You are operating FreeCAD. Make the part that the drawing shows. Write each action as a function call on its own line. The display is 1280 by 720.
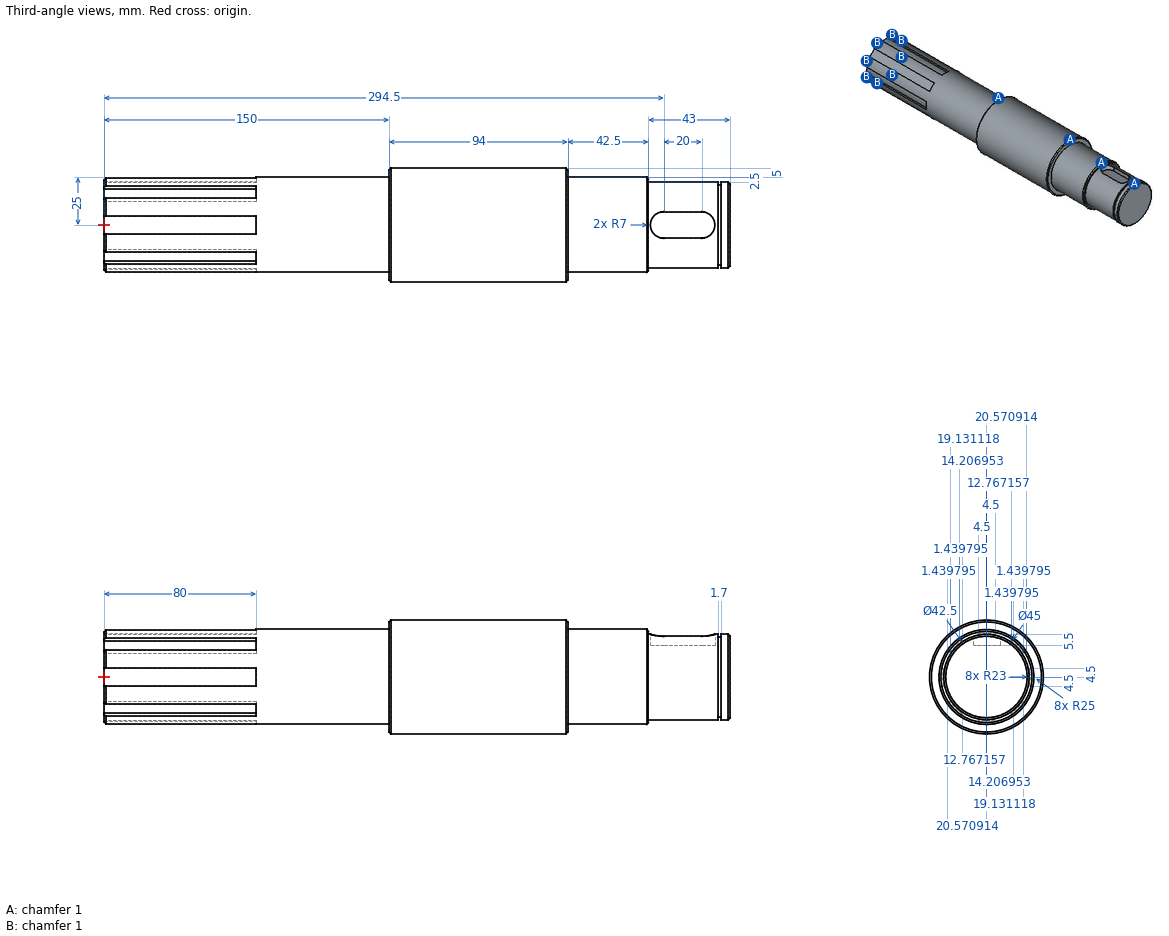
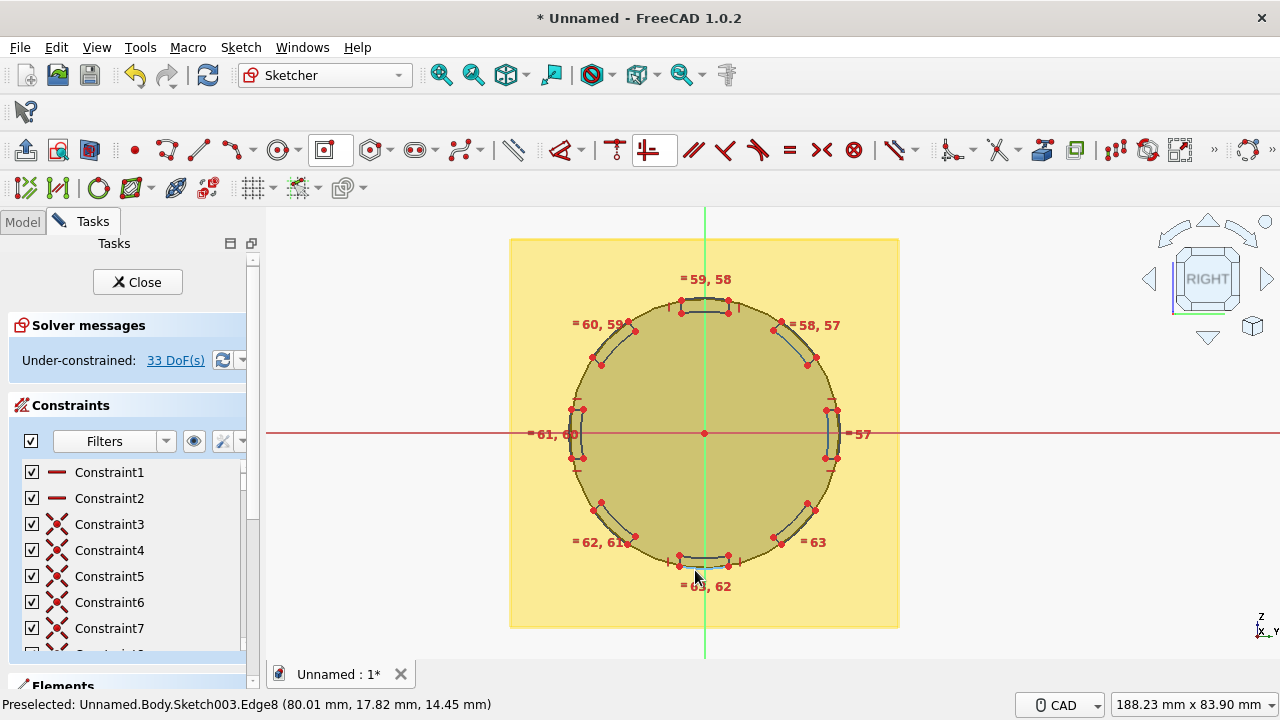
scroll(714, 312, up, 2)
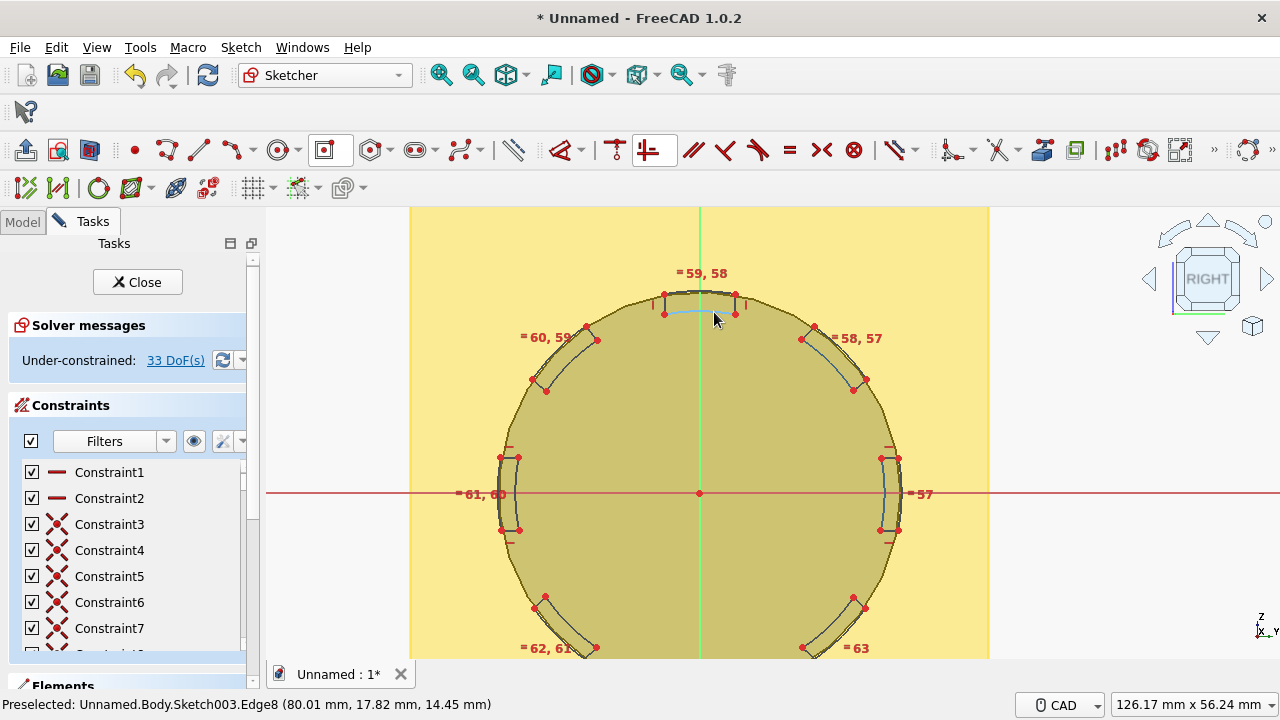
click(714, 312)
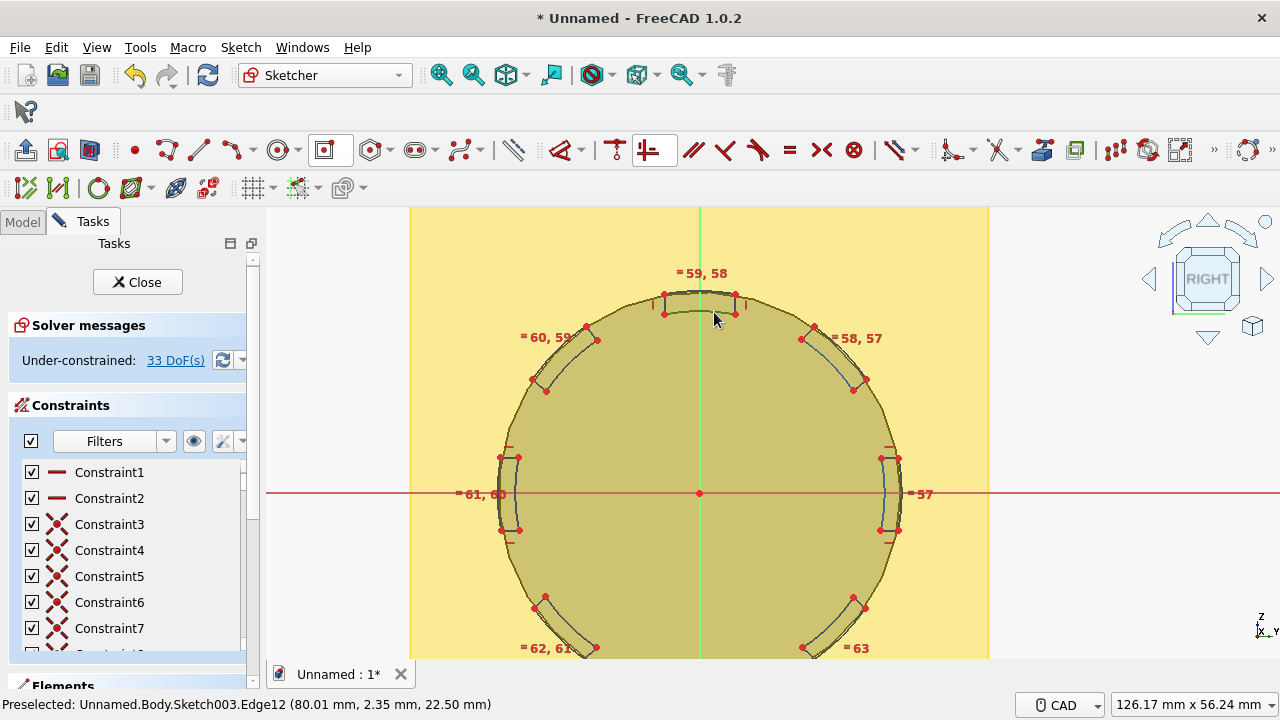
click(580, 354)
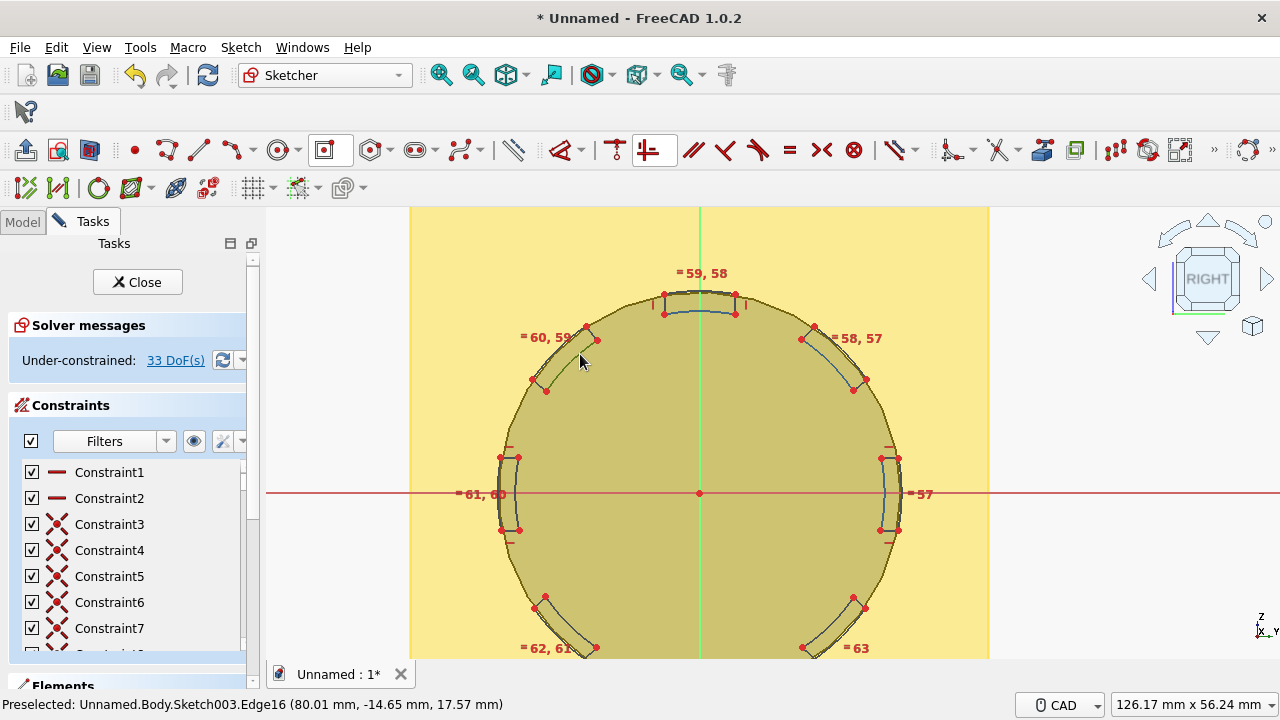
click(516, 480)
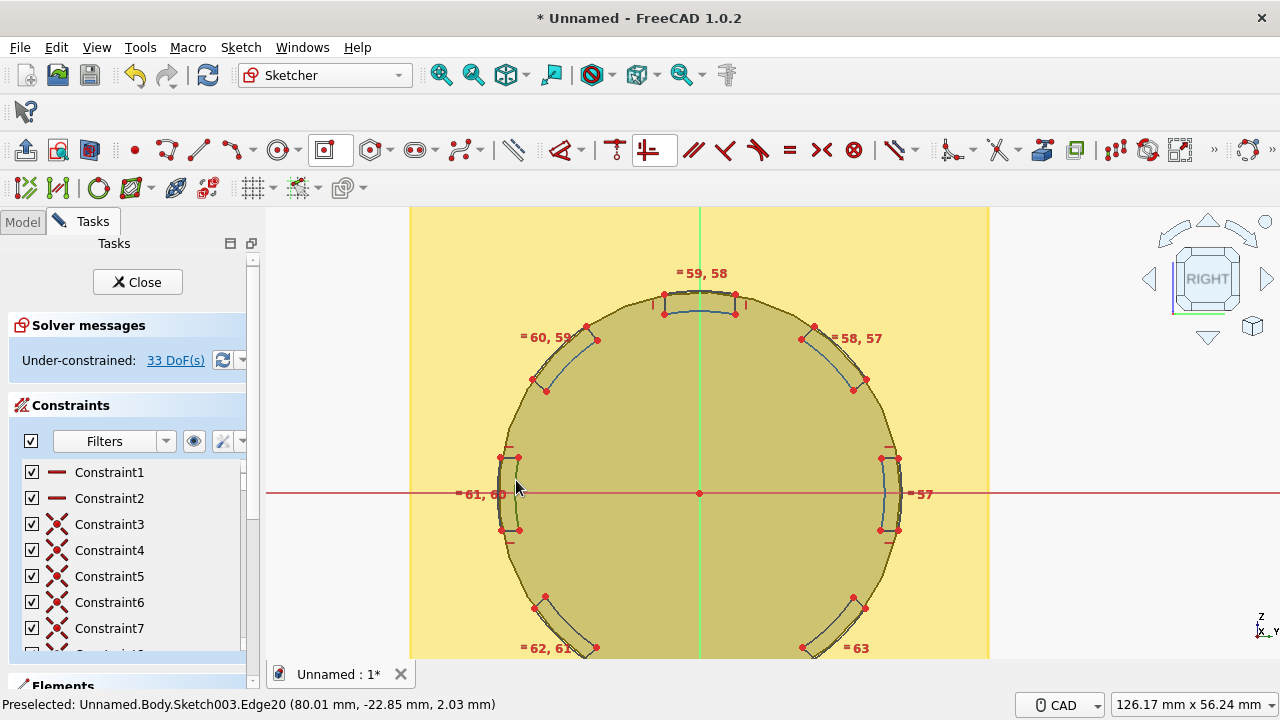
click(559, 614)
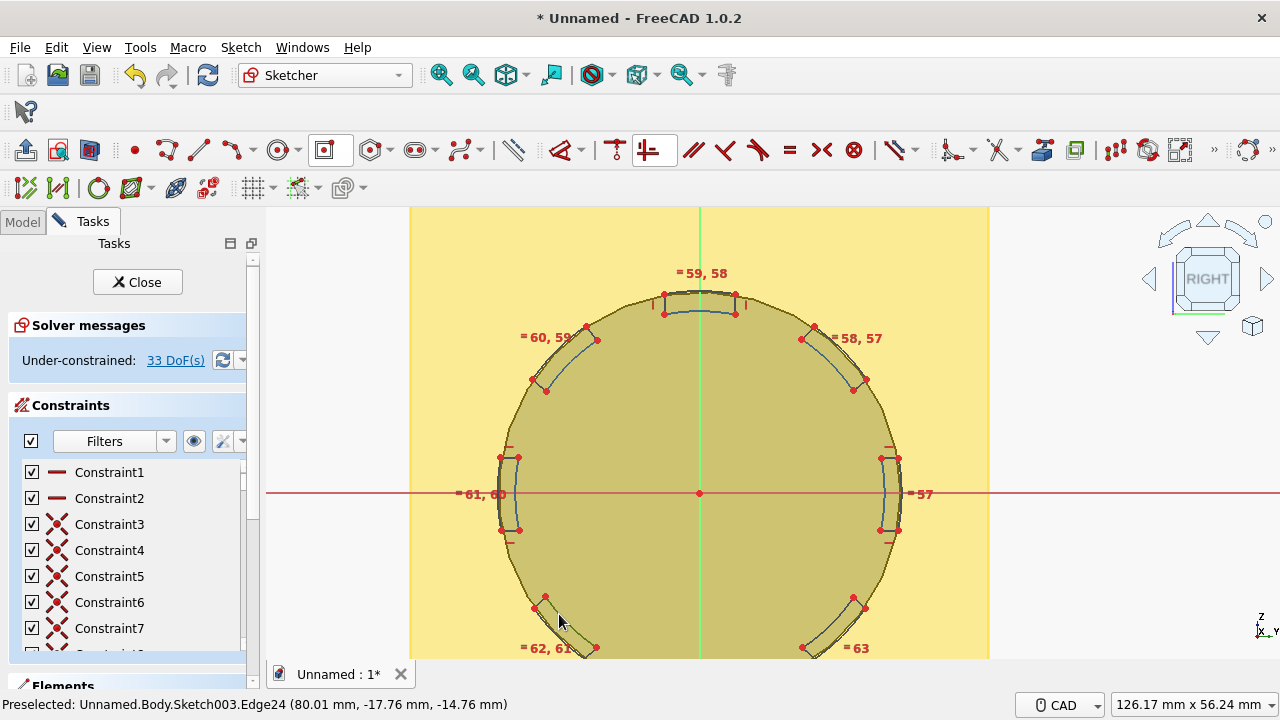
scroll(714, 311, down, 2)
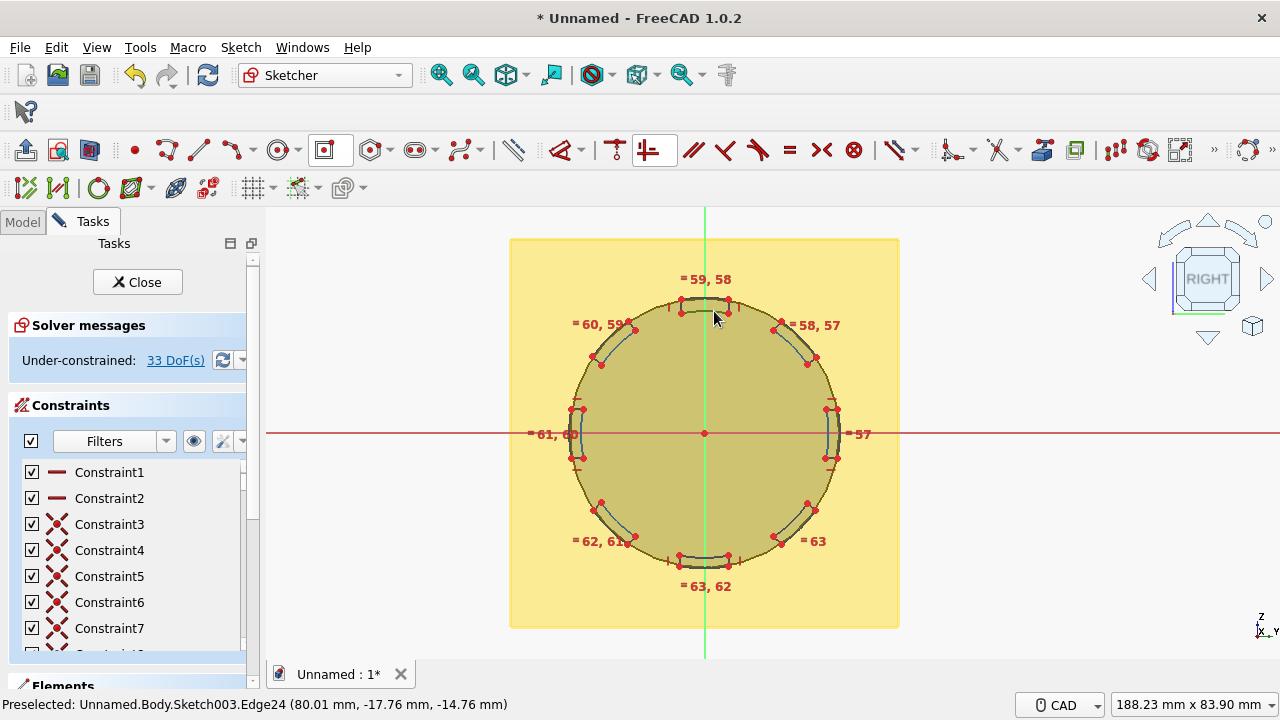
scroll(695, 557, up, 2)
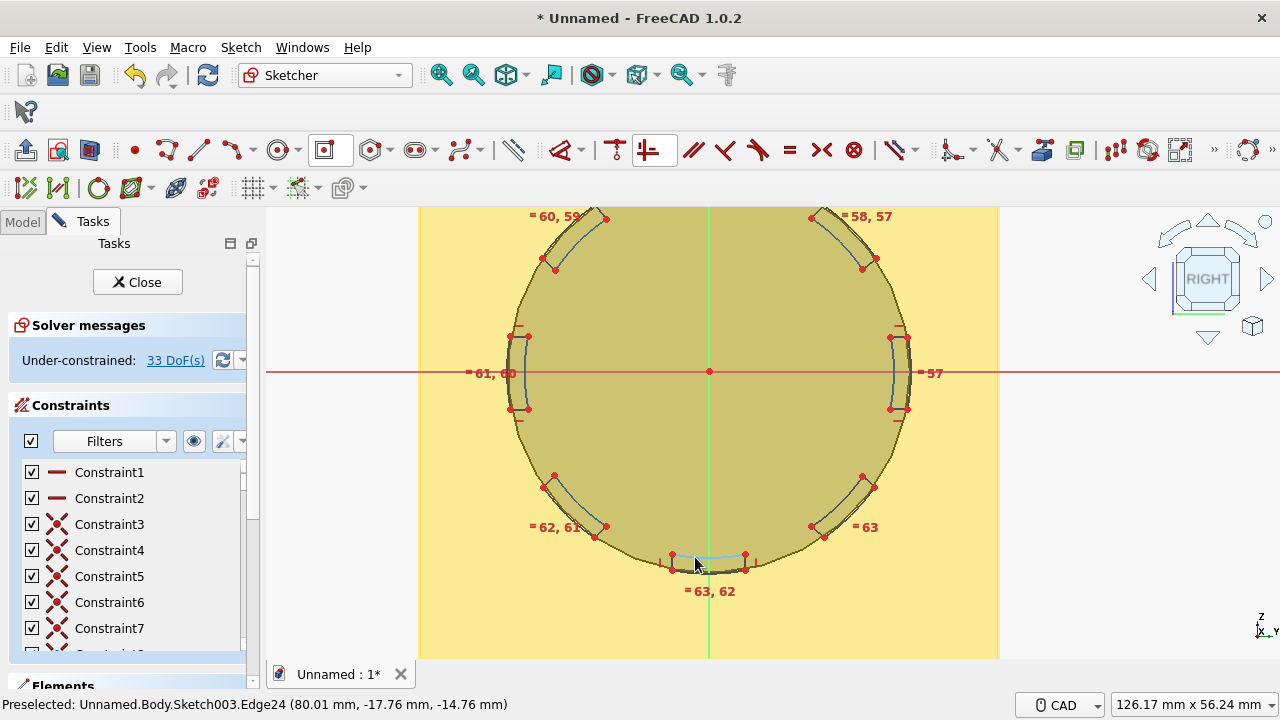
click(694, 557)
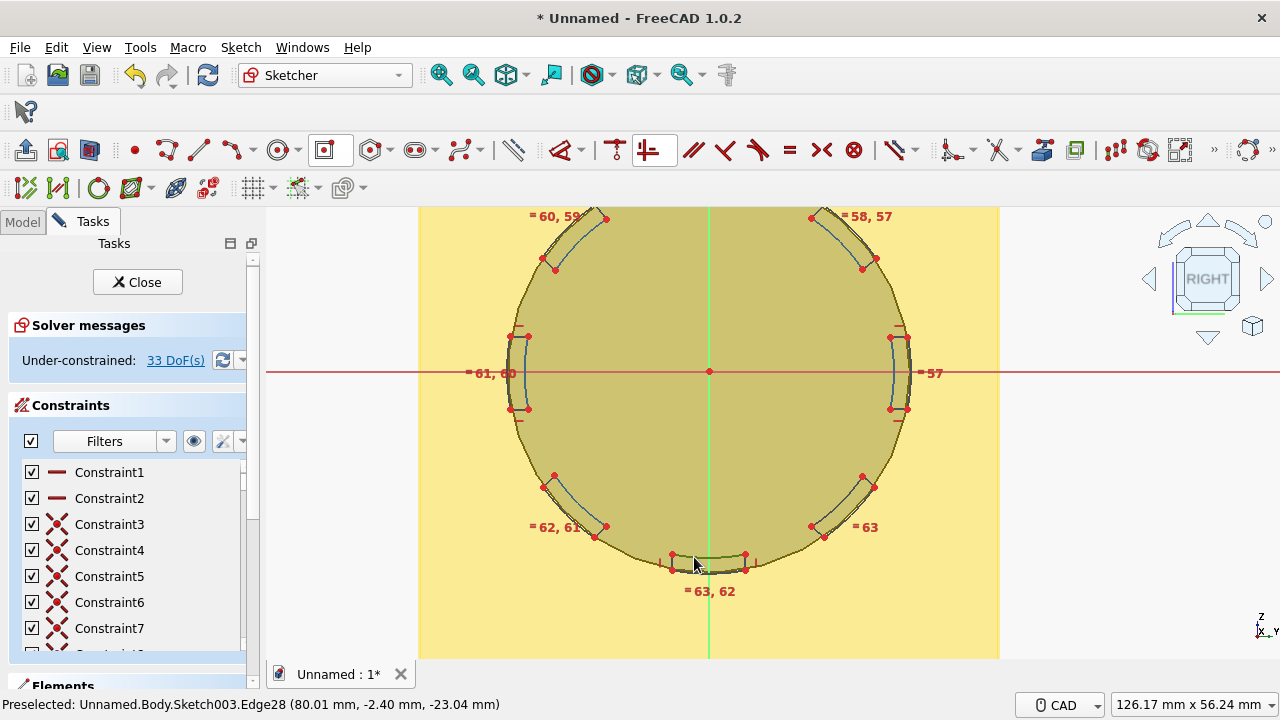
click(829, 514)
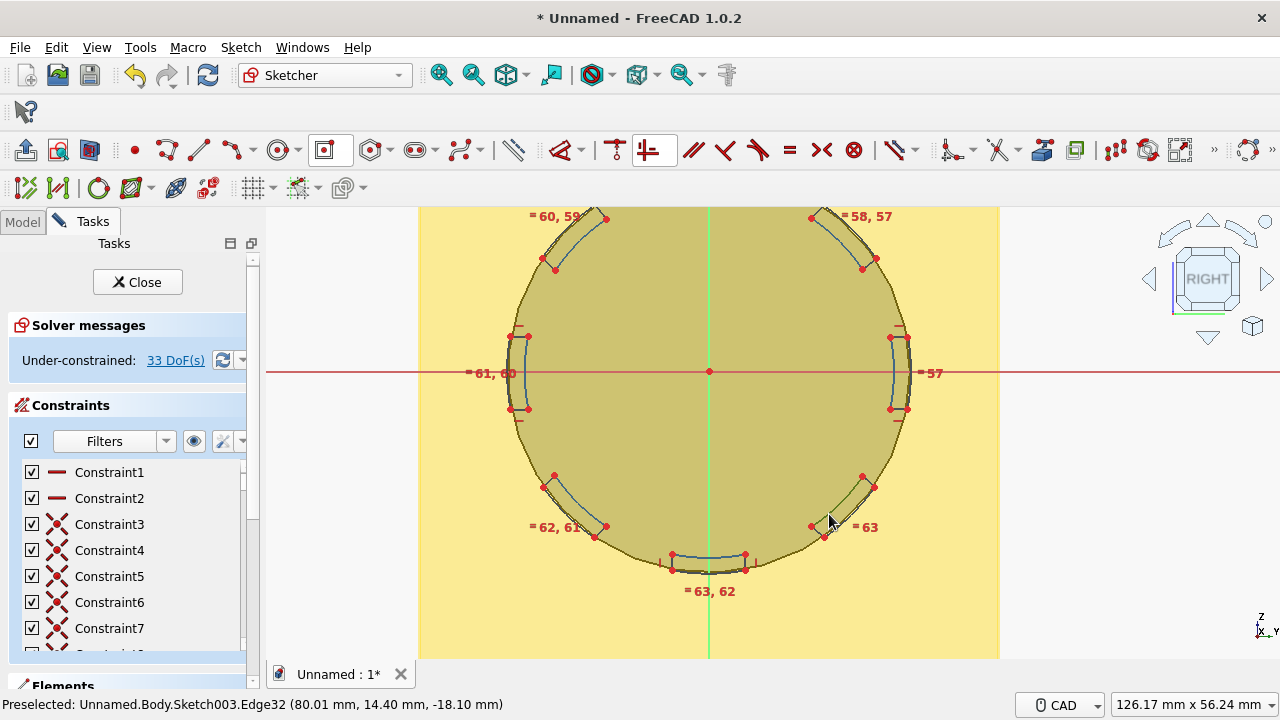
click(790, 150)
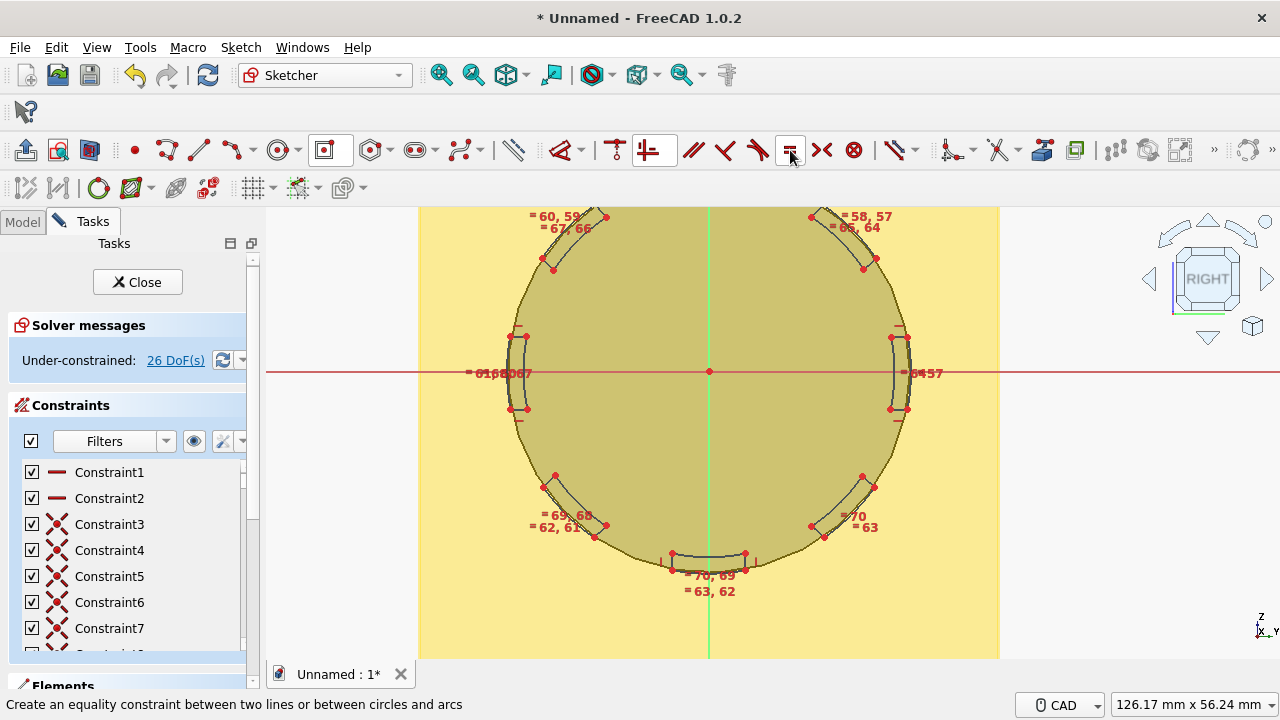
click(560, 150)